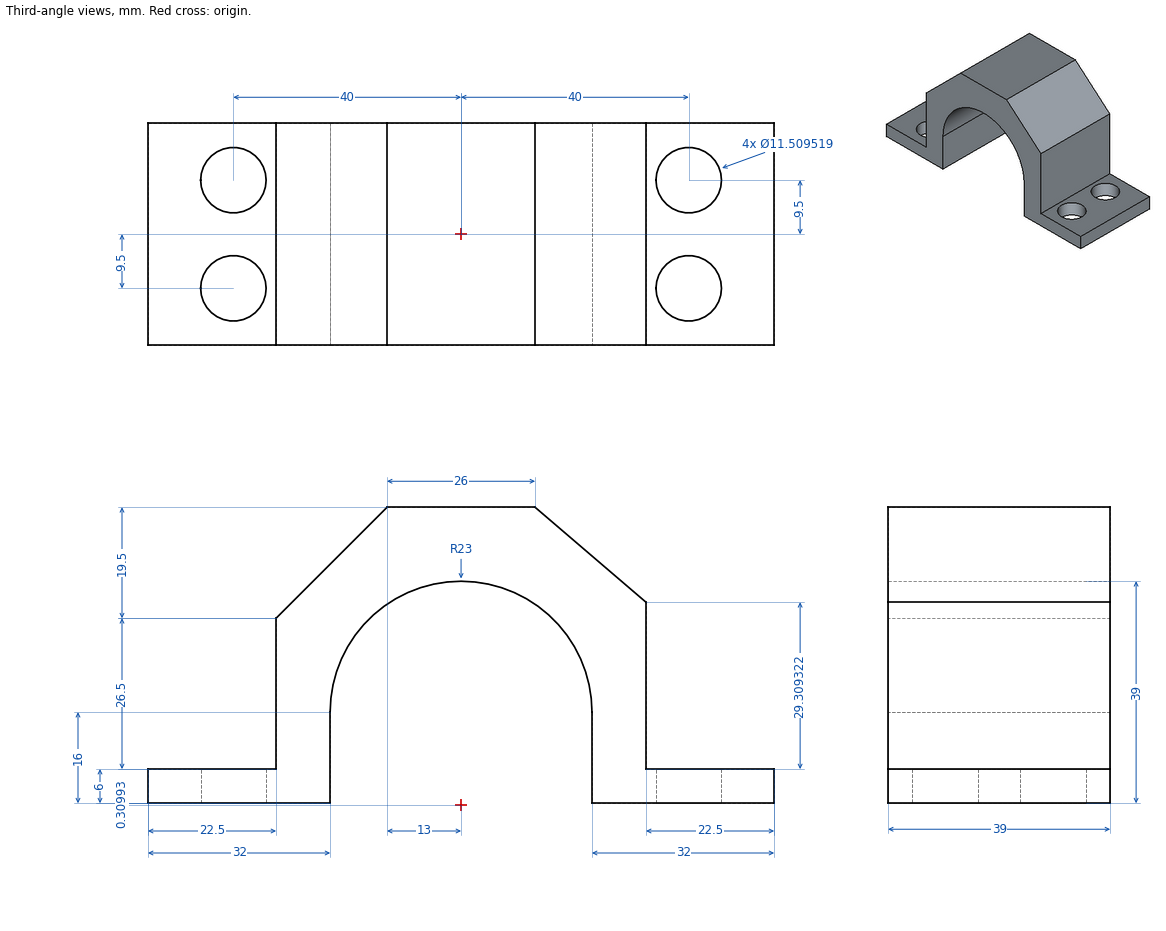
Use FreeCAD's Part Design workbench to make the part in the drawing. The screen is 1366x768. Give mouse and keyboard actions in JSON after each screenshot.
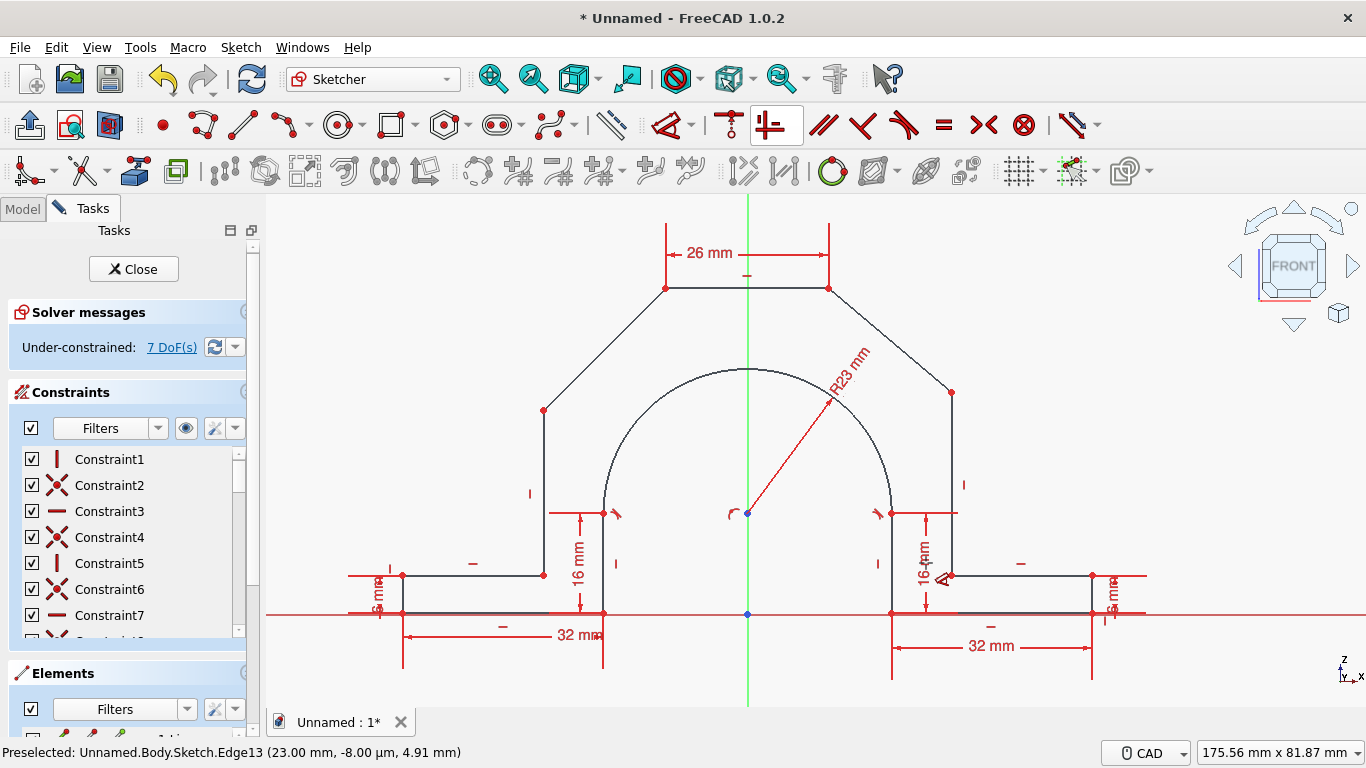
{"action": "left_click", "coordinate": [666, 288]}
{"action": "left_click", "coordinate": [707, 649]}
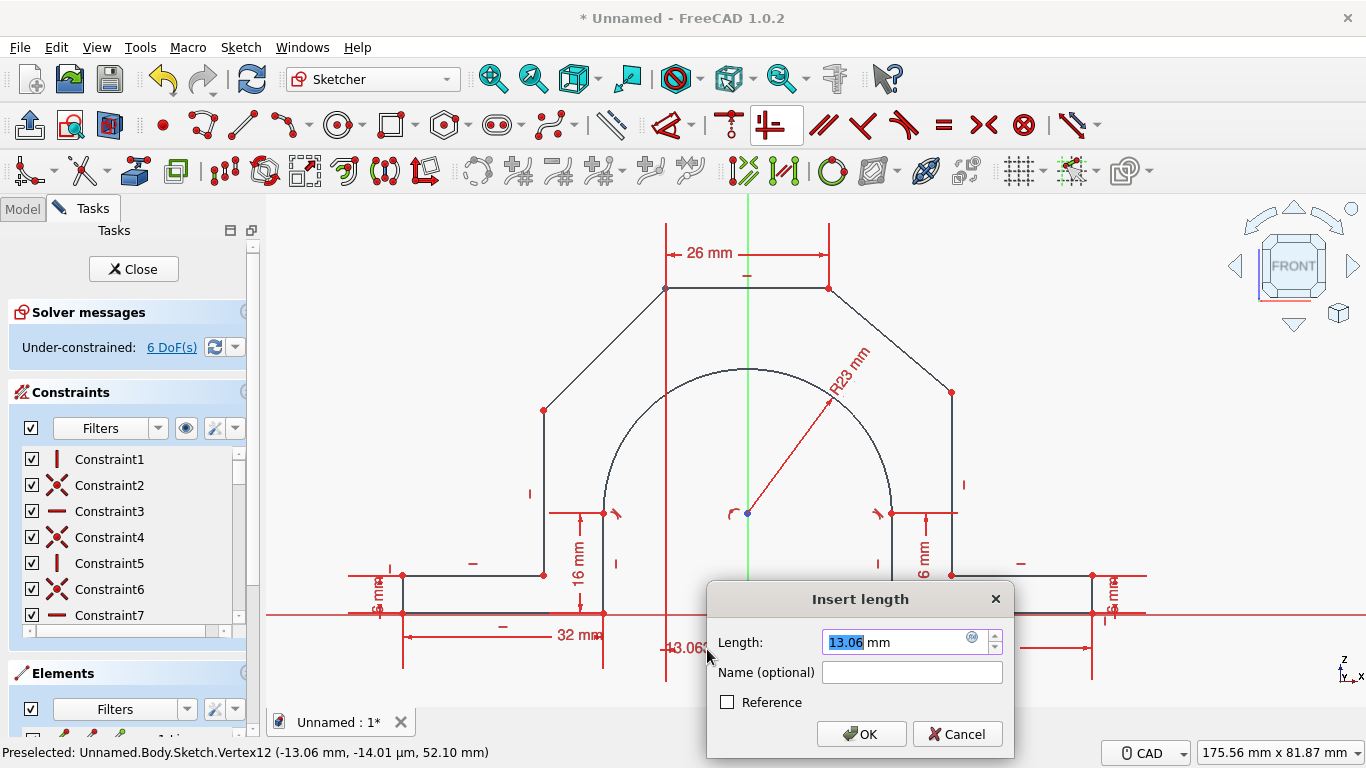
{"action": "type", "text": "13"}
{"action": "key", "text": "Return"}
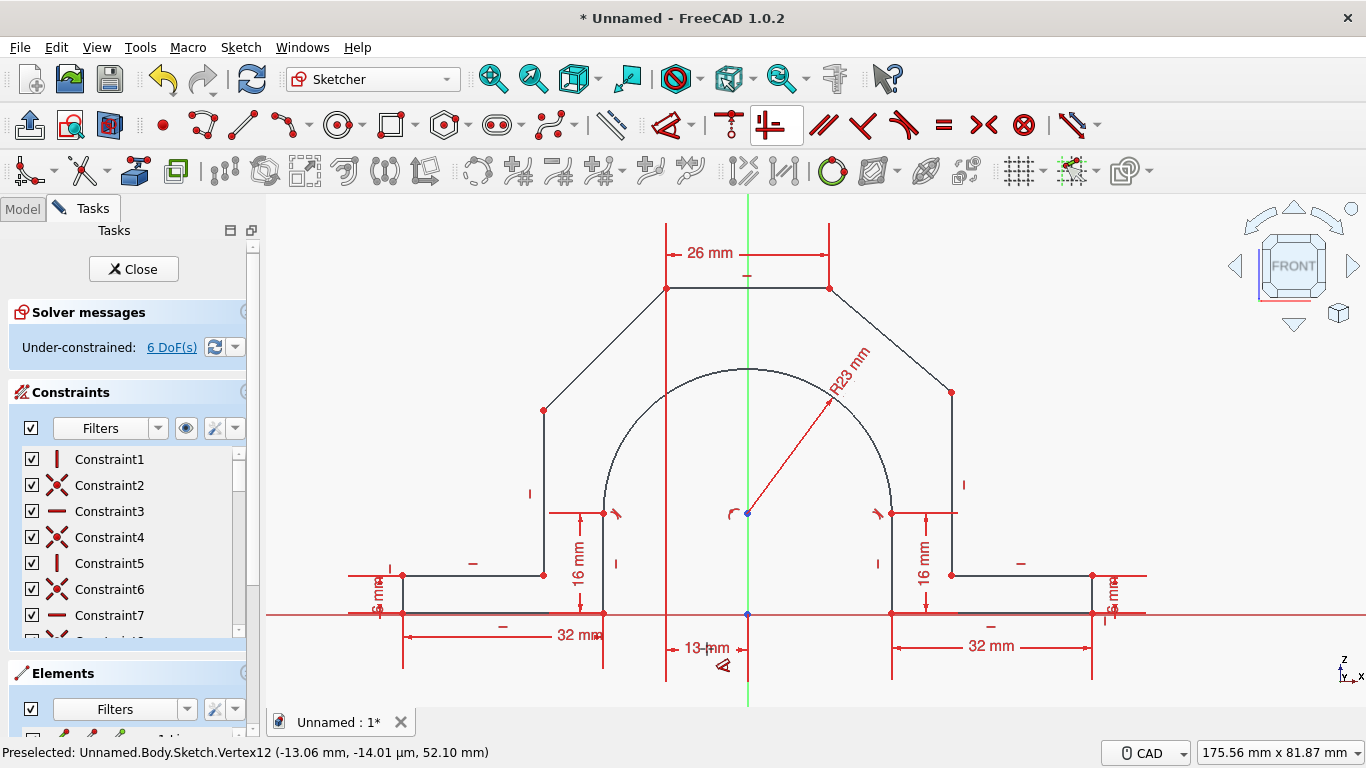
{"action": "left_click", "coordinate": [445, 576]}
{"action": "left_click", "coordinate": [473, 542]}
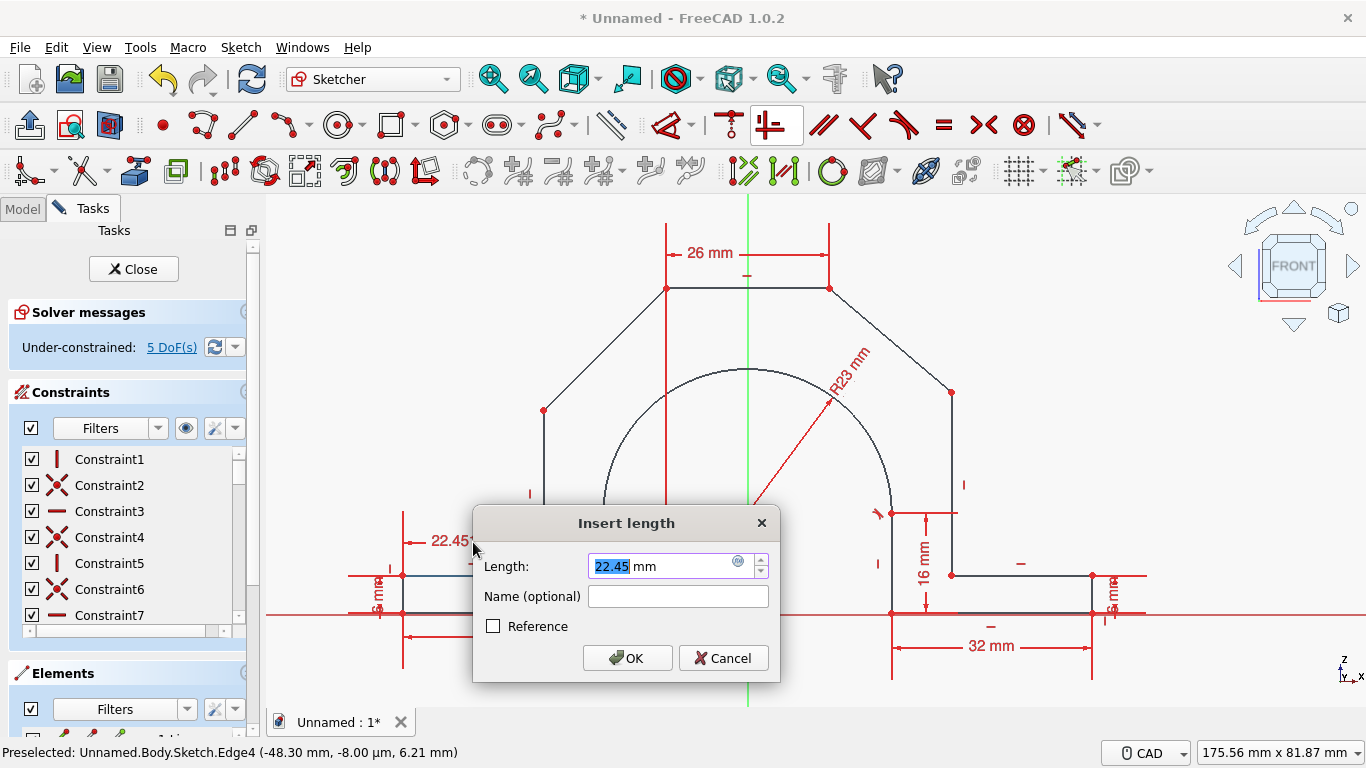
{"action": "type", "text": "22.5"}
{"action": "key", "text": "Return"}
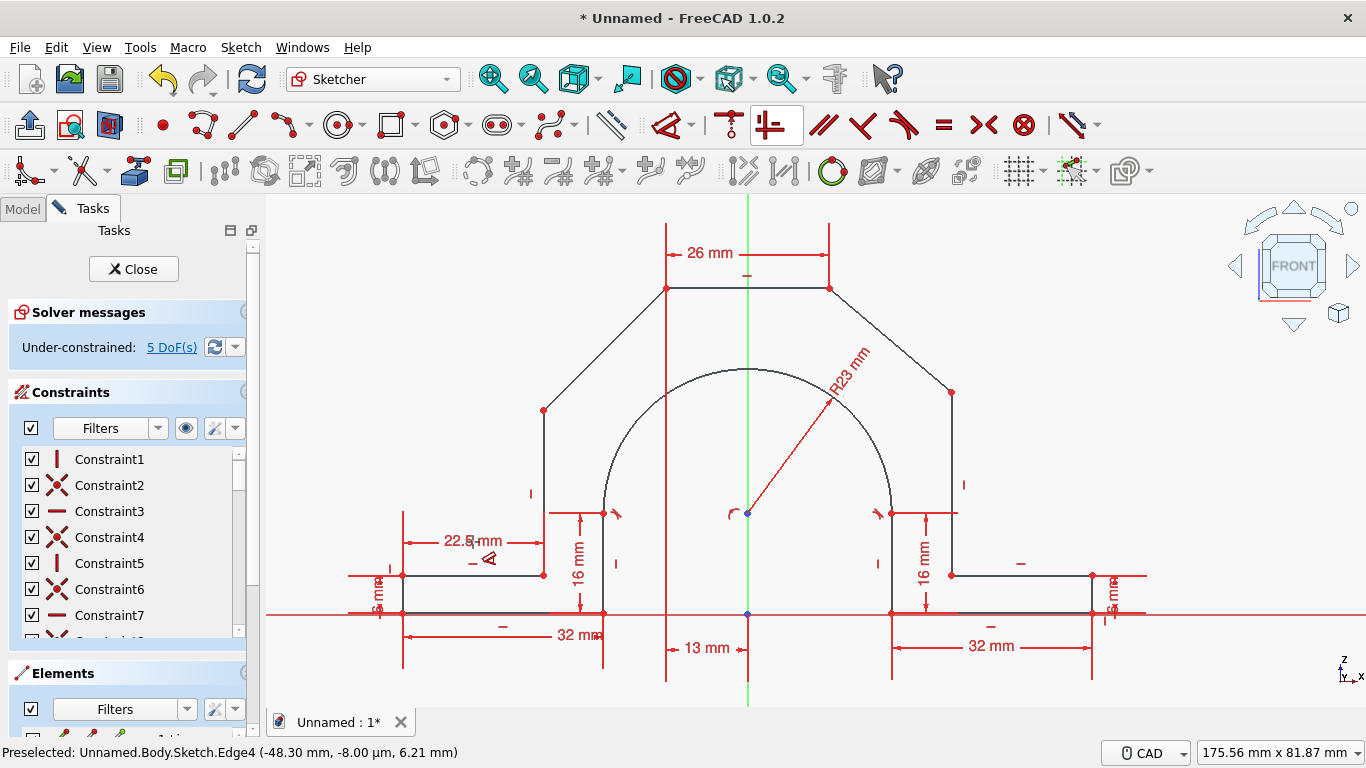
{"action": "left_click", "coordinate": [544, 526]}
{"action": "left_click", "coordinate": [510, 493]}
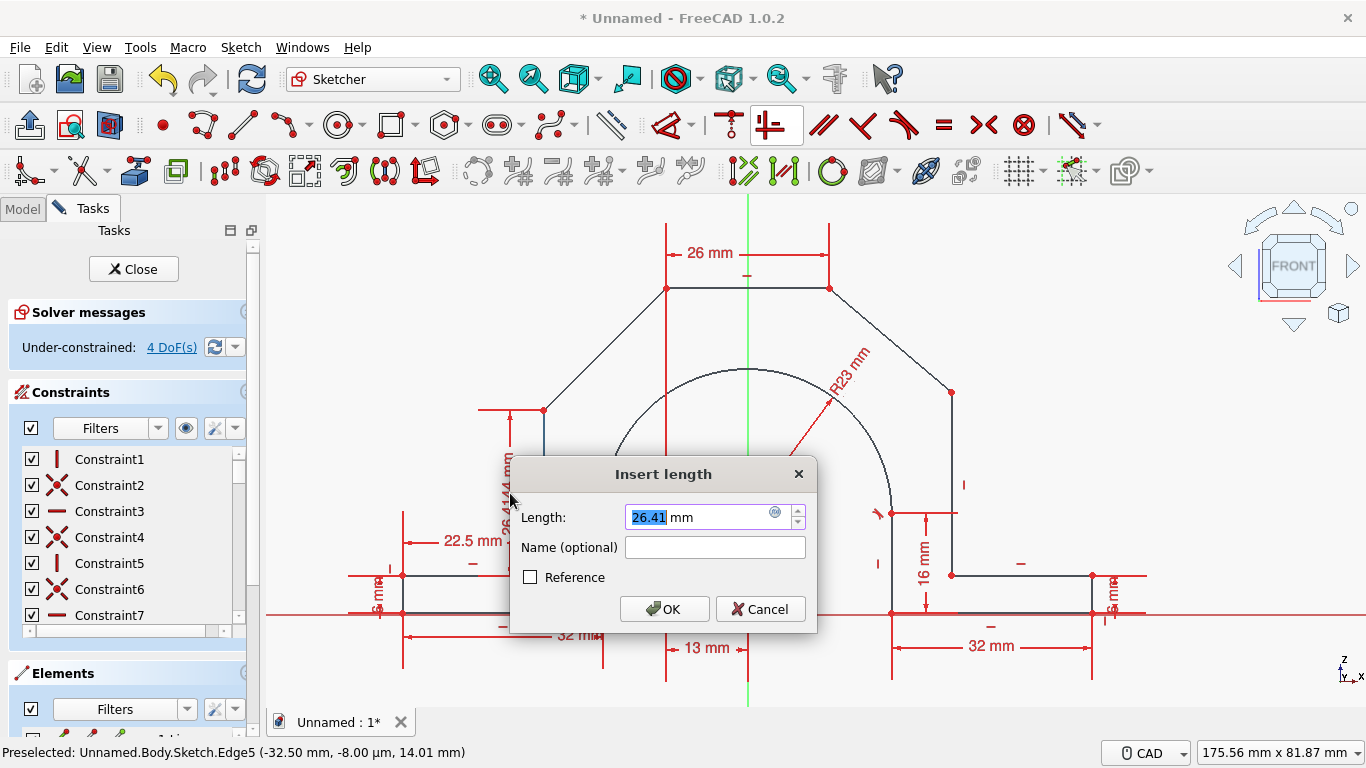
{"action": "type", "text": "26.5"}
{"action": "key", "text": "Return"}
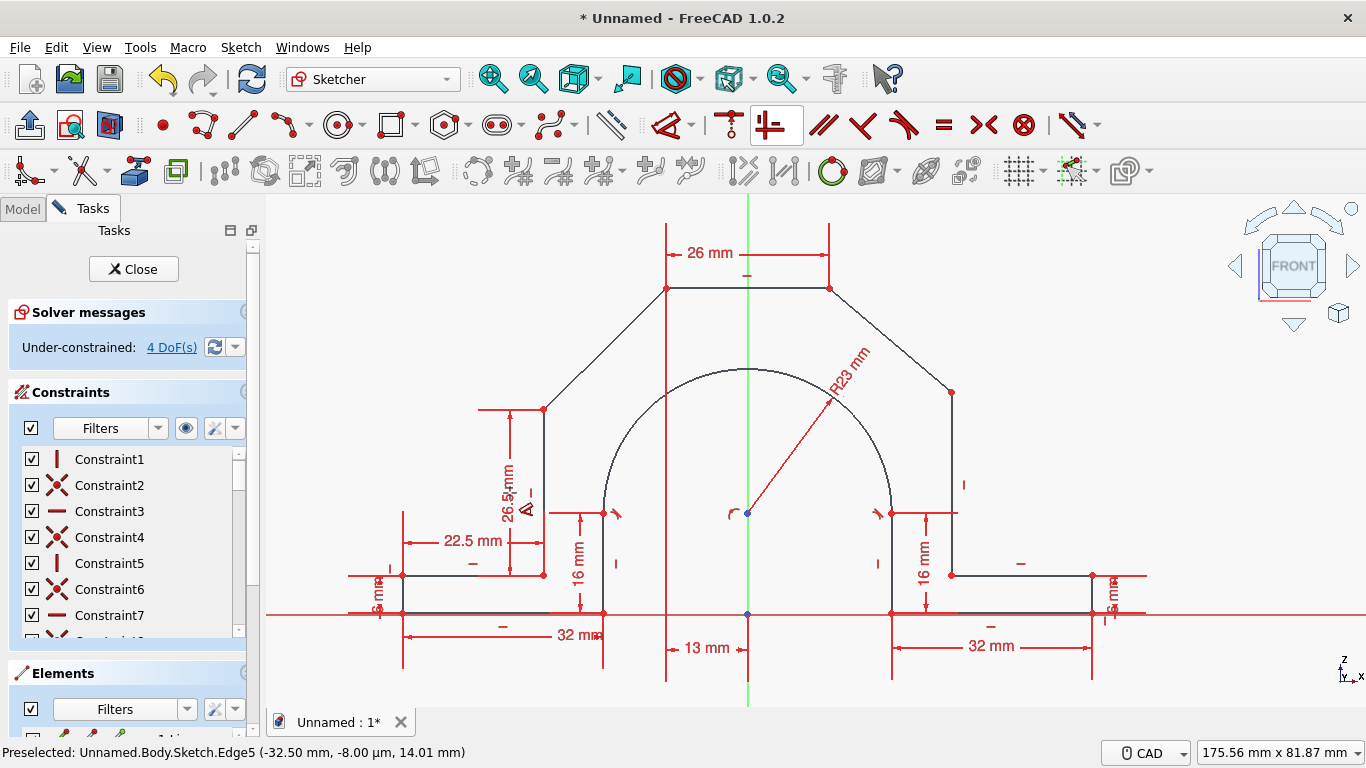
{"action": "left_click", "coordinate": [994, 576]}
{"action": "left_click", "coordinate": [1022, 542]}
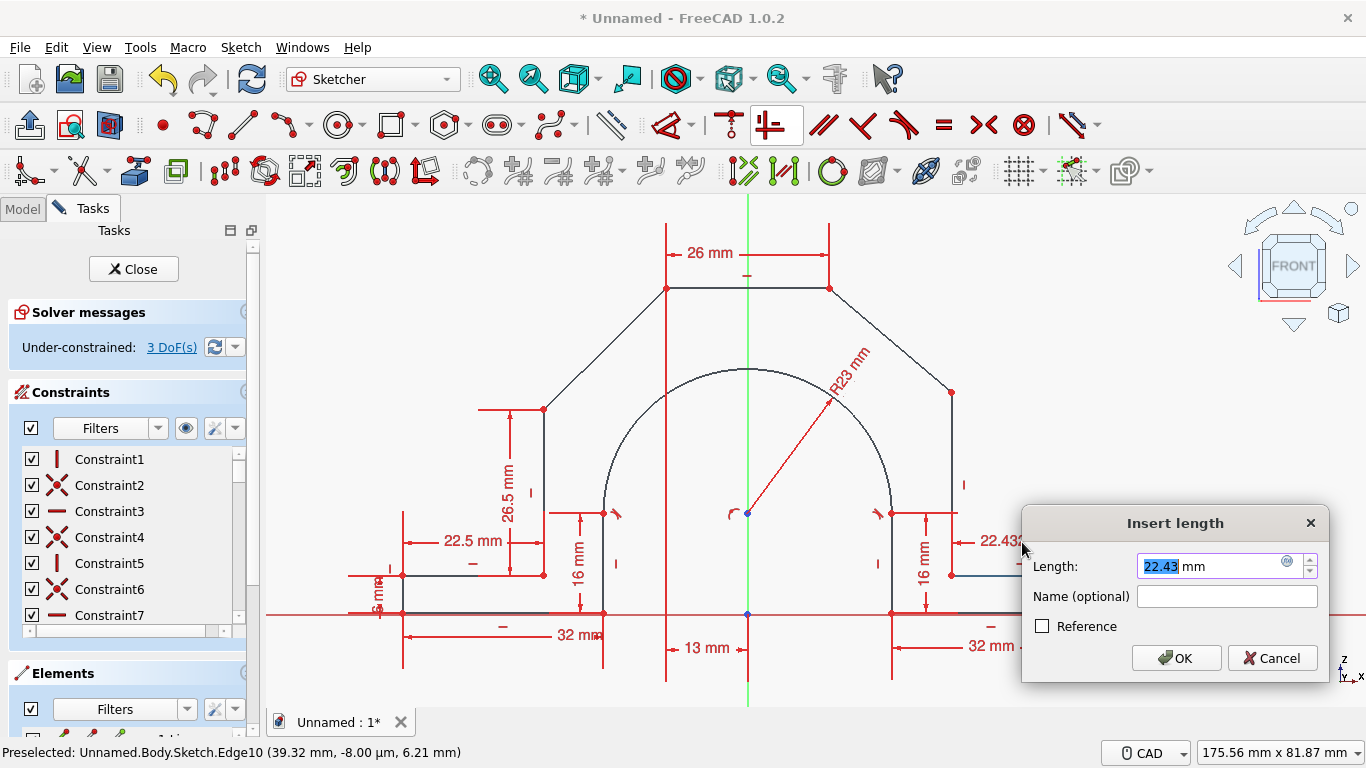
{"action": "type", "text": "22.5"}
{"action": "key", "text": "Return"}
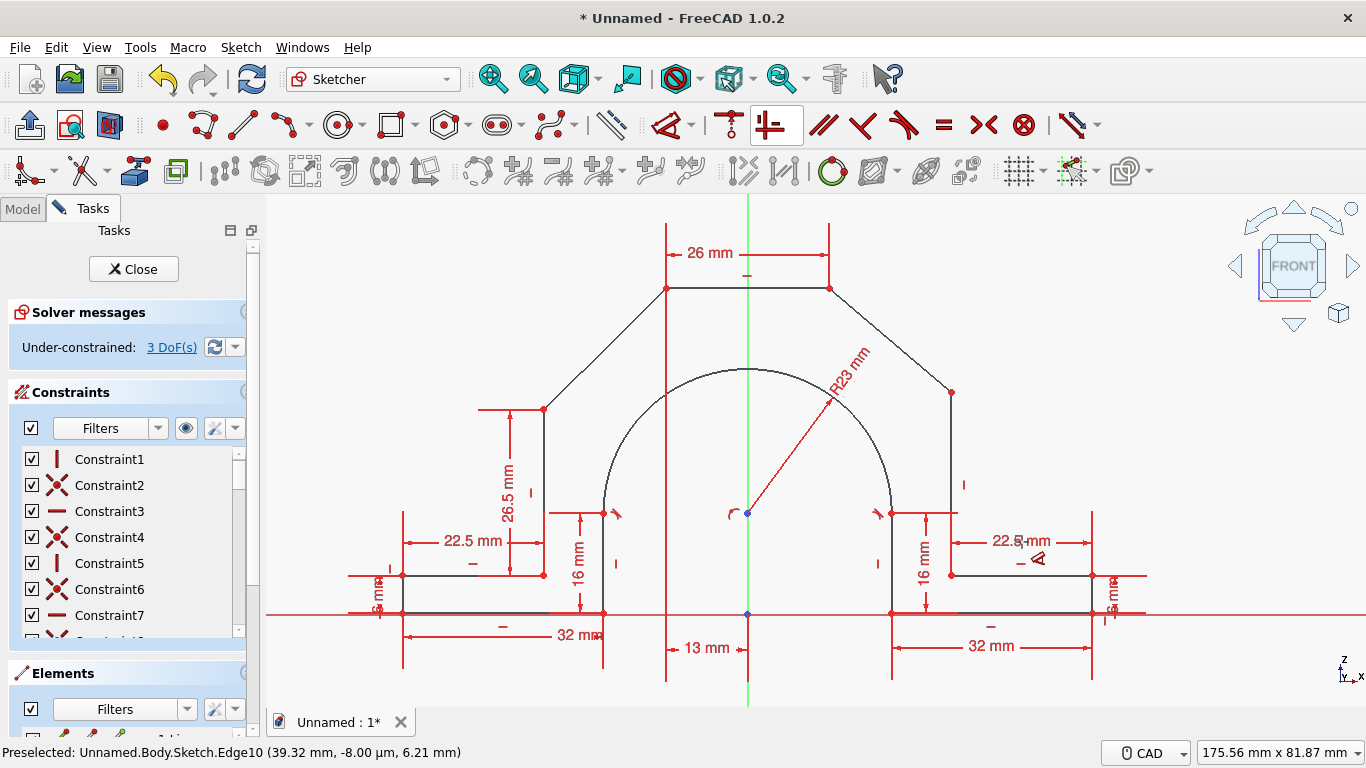
{"action": "left_click", "coordinate": [581, 373]}
{"action": "left_click", "coordinate": [510, 349]}